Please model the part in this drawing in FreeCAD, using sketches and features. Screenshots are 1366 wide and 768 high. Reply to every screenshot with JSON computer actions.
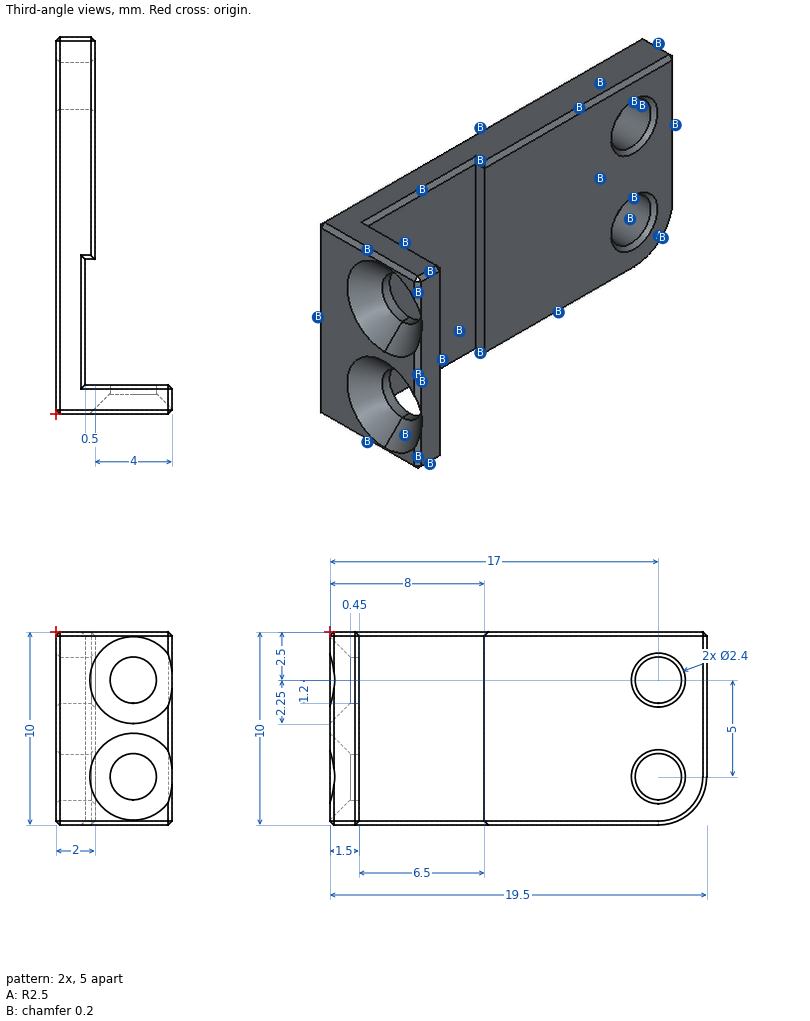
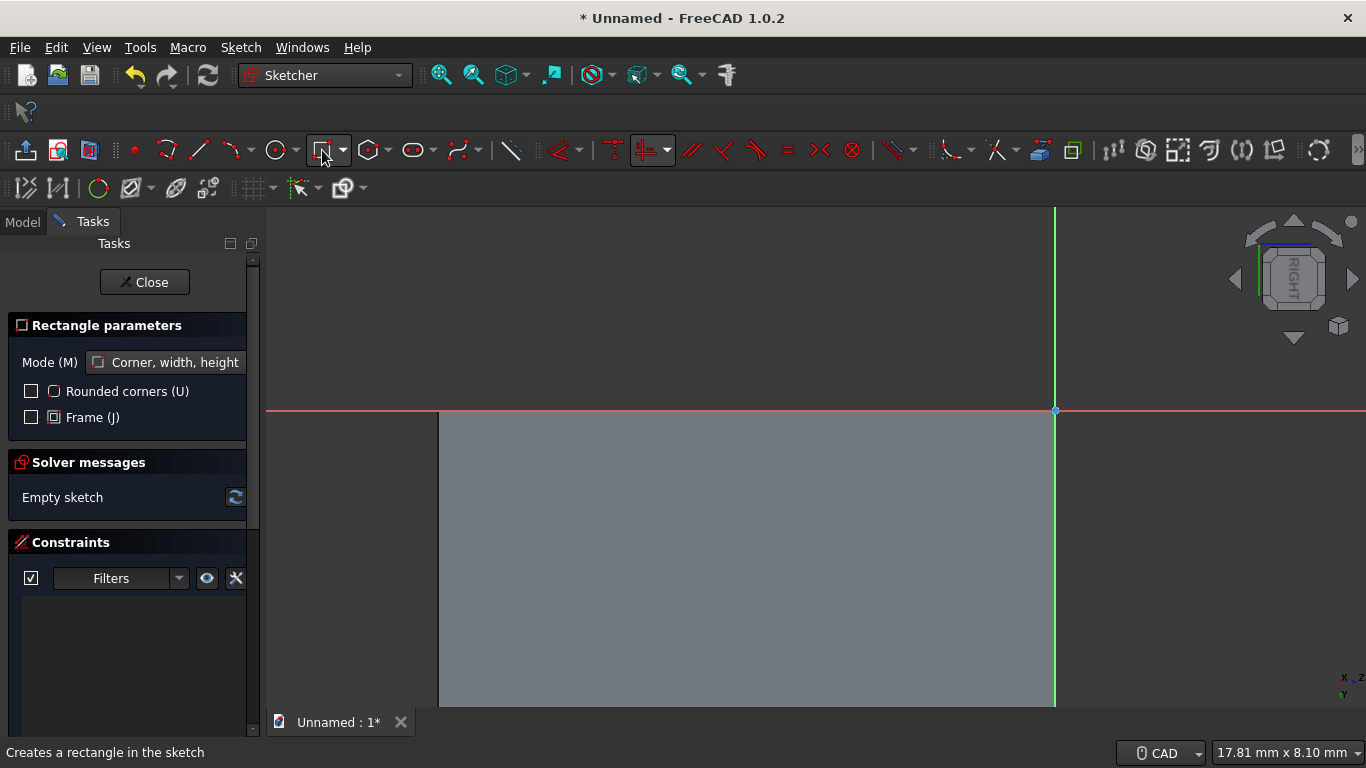
{"action": "left_click", "coordinate": [1055, 411]}
{"action": "left_click", "coordinate": [438, 504]}
{"action": "key", "text": "Escape"}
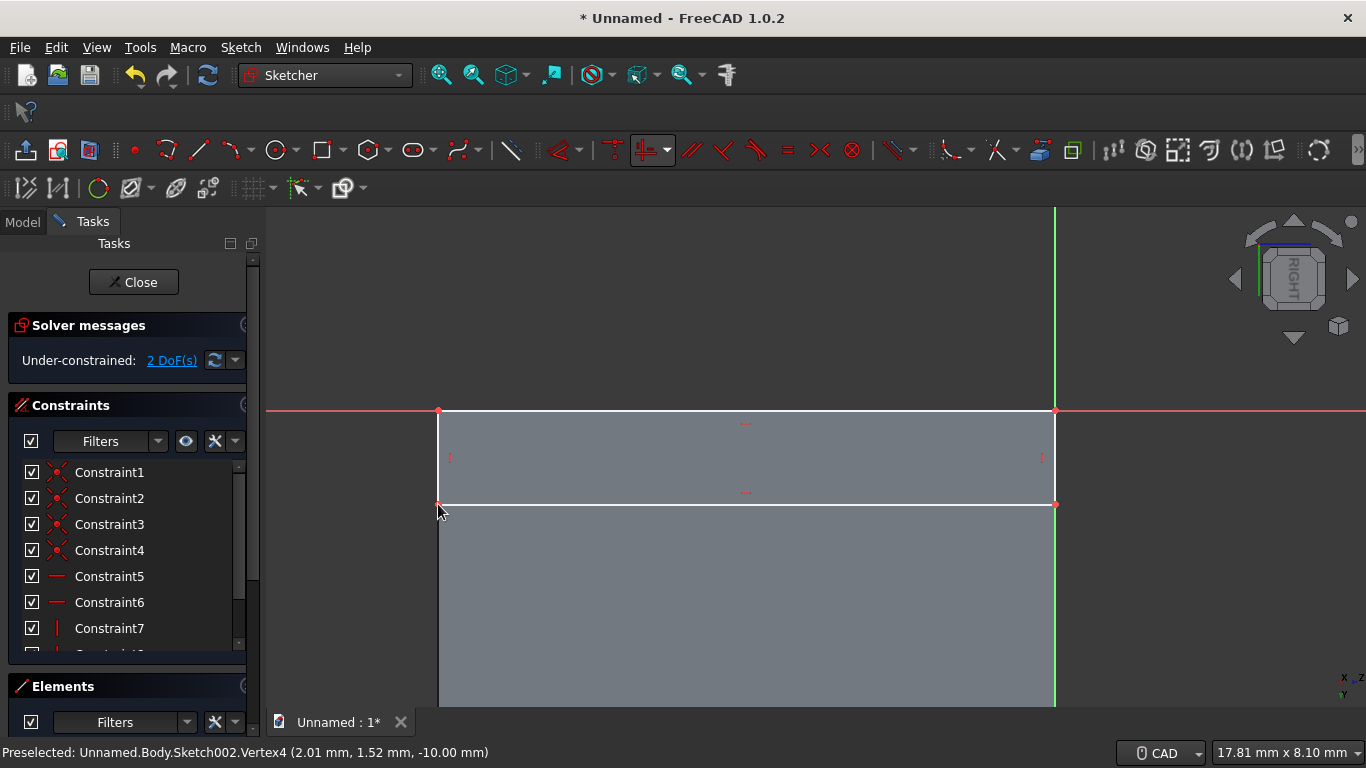
{"action": "left_click", "coordinate": [558, 150]}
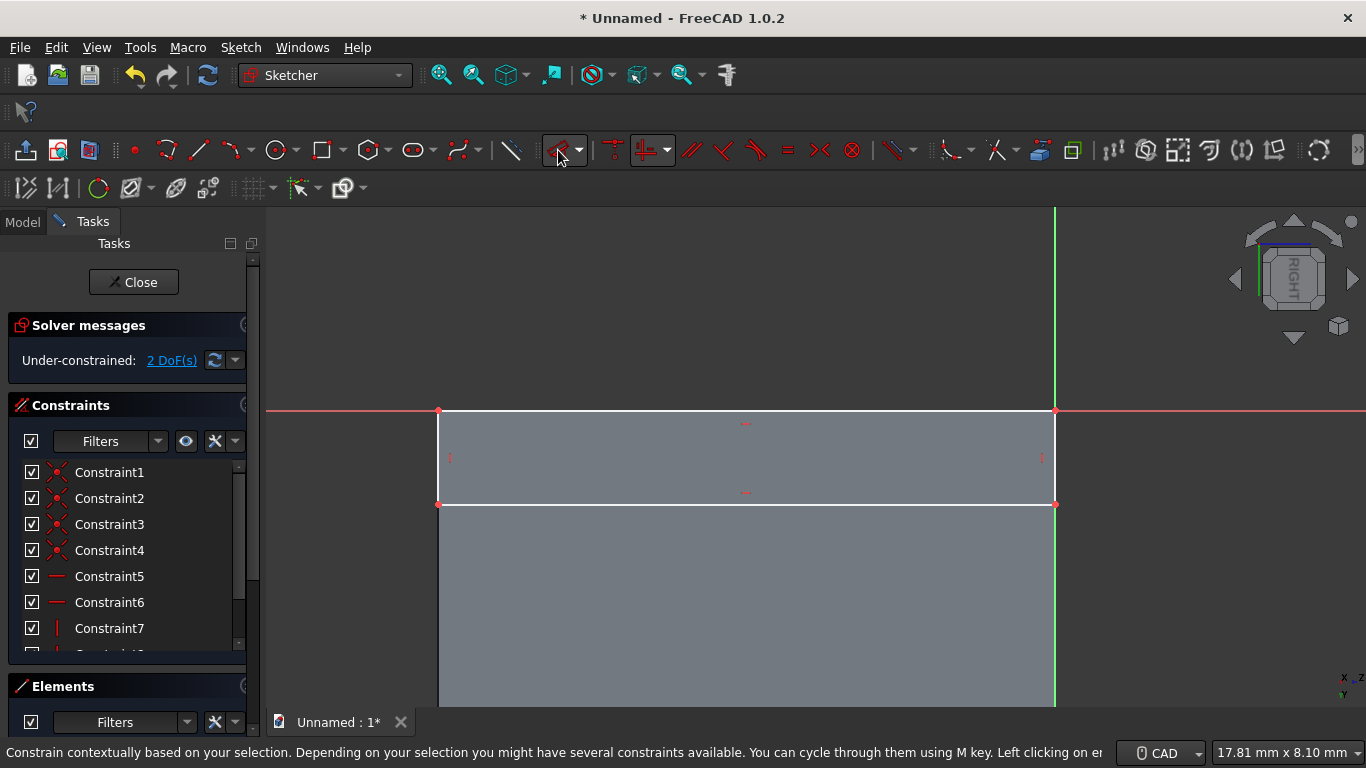
{"action": "left_click", "coordinate": [870, 411]}
{"action": "left_click", "coordinate": [747, 377]}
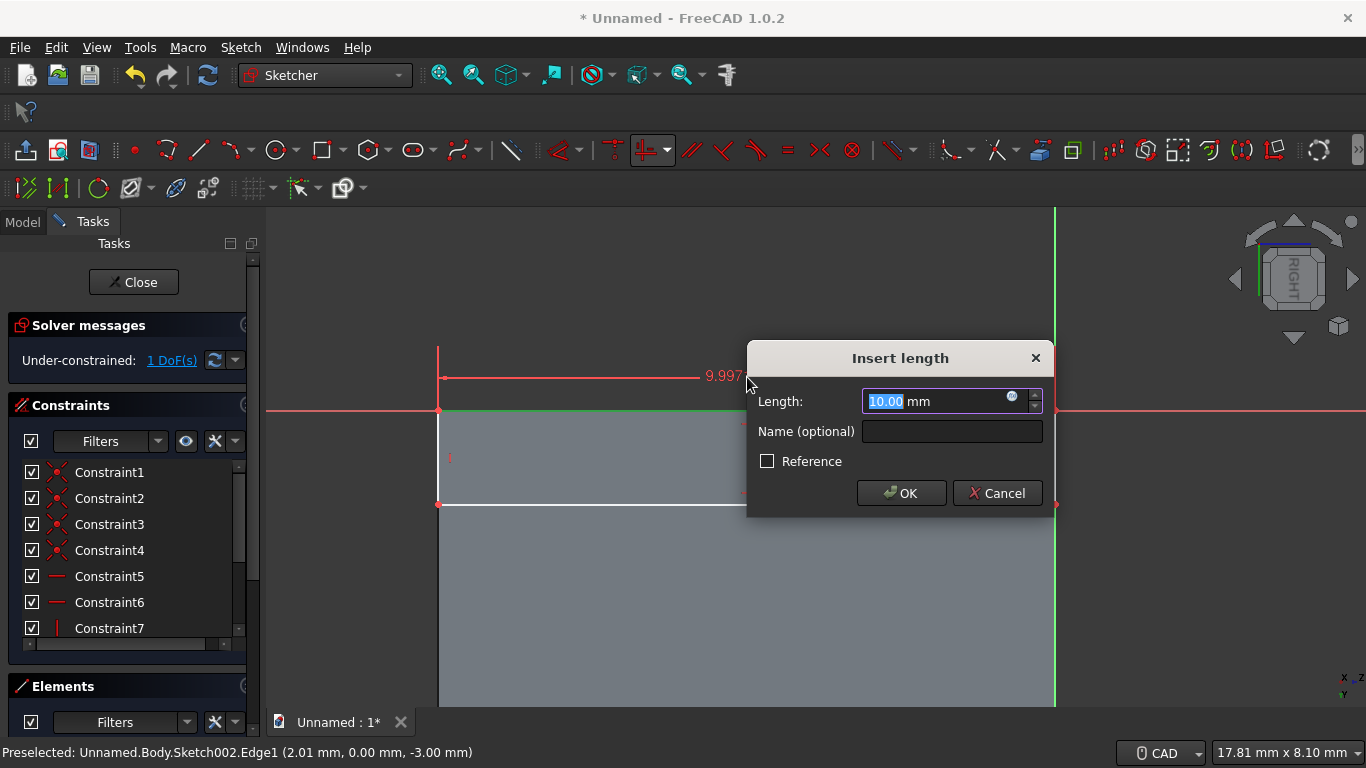
{"action": "type", "text": "10"}
{"action": "key", "text": "Return"}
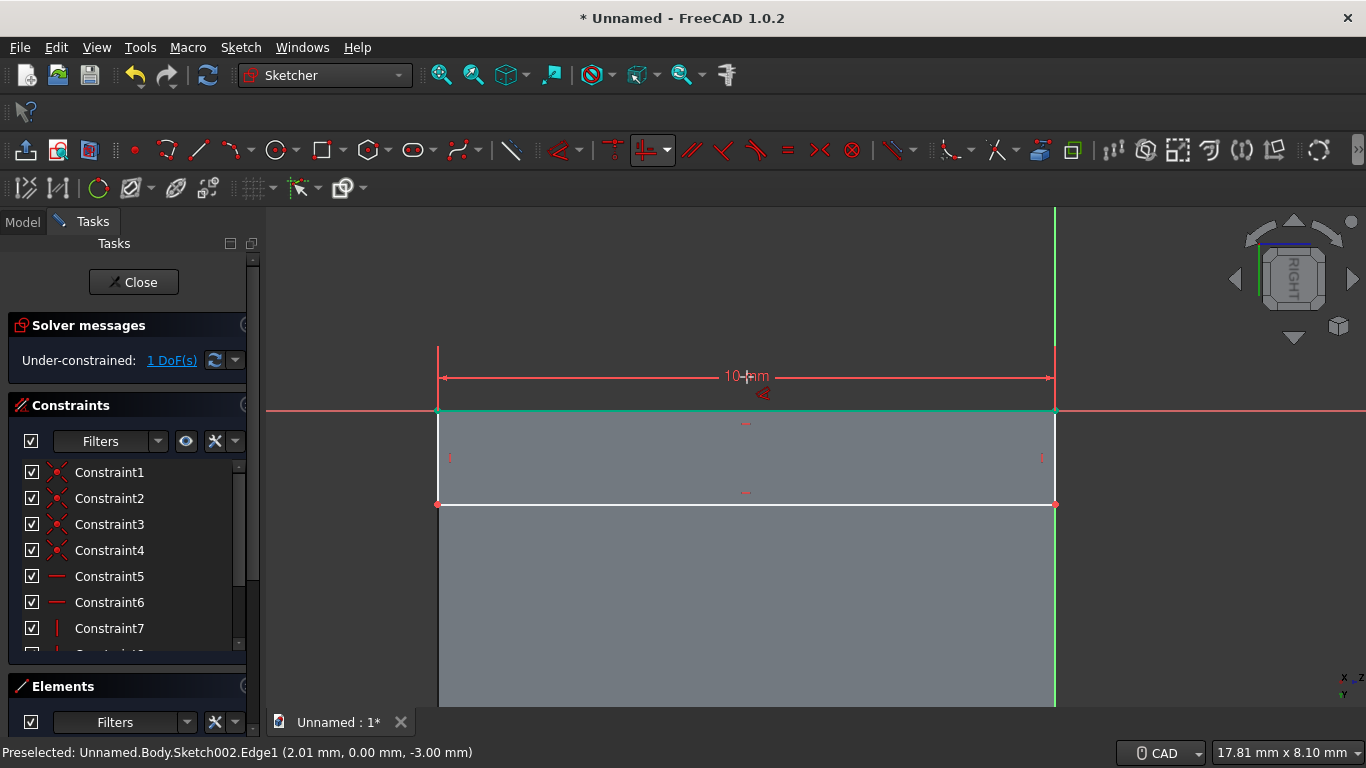
{"action": "left_click", "coordinate": [438, 439]}
{"action": "left_click", "coordinate": [404, 458]}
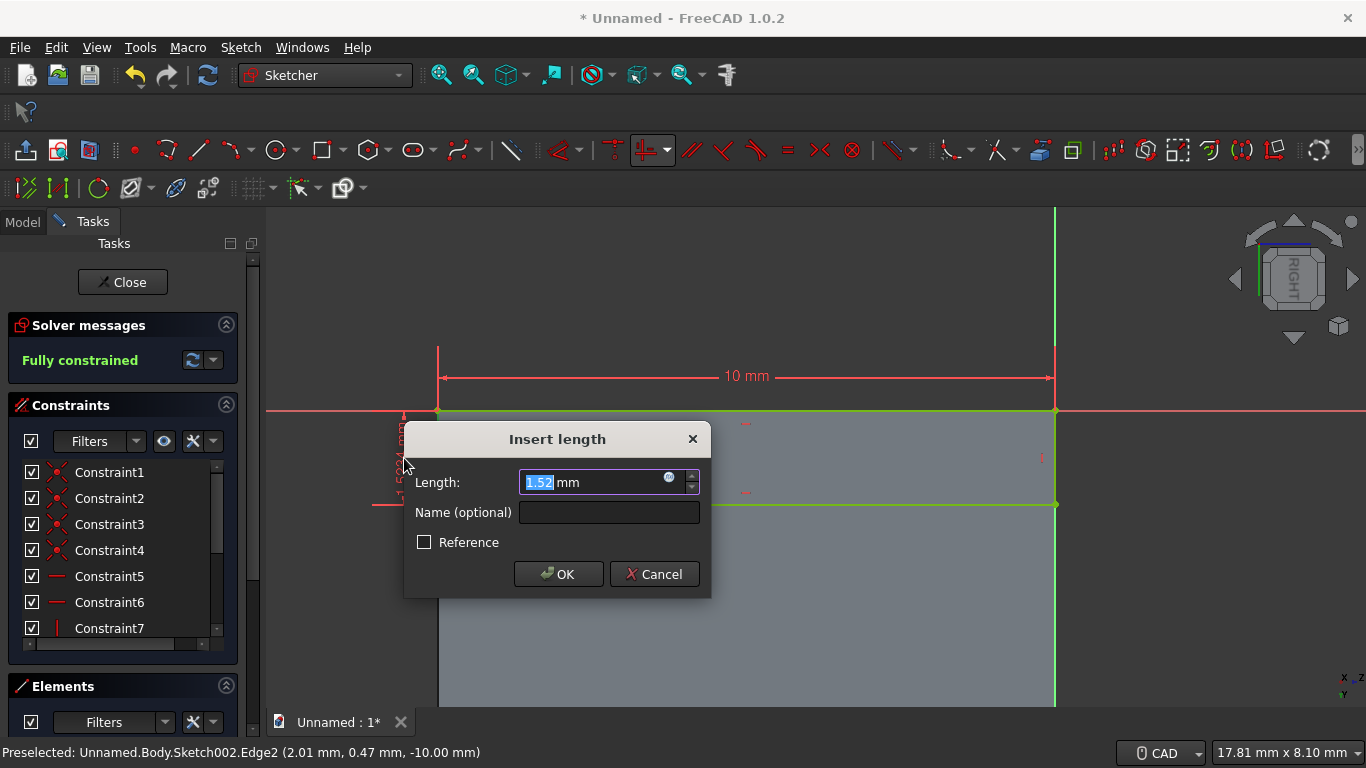
{"action": "type", "text": "1.5"}
{"action": "key", "text": "Return"}
{"action": "key", "text": "Escape"}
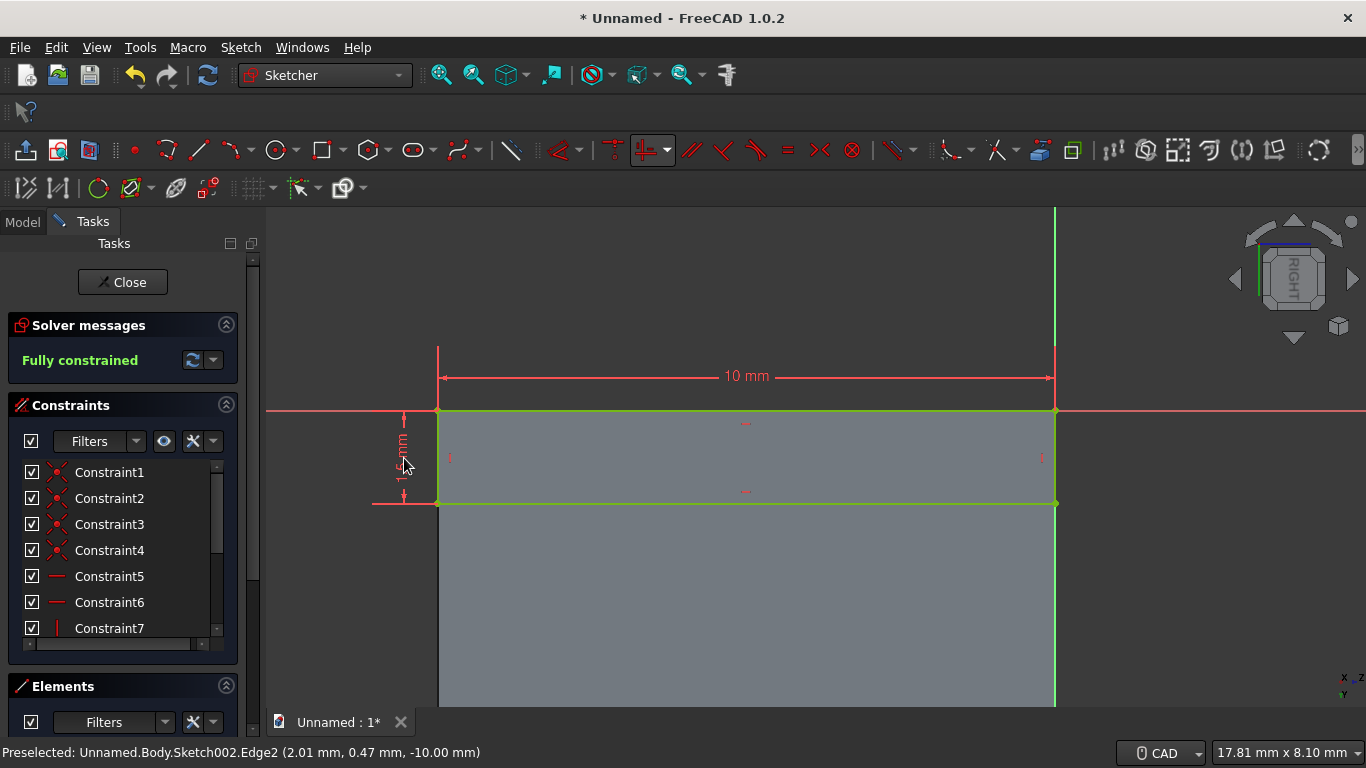
{"action": "left_click", "coordinate": [123, 282]}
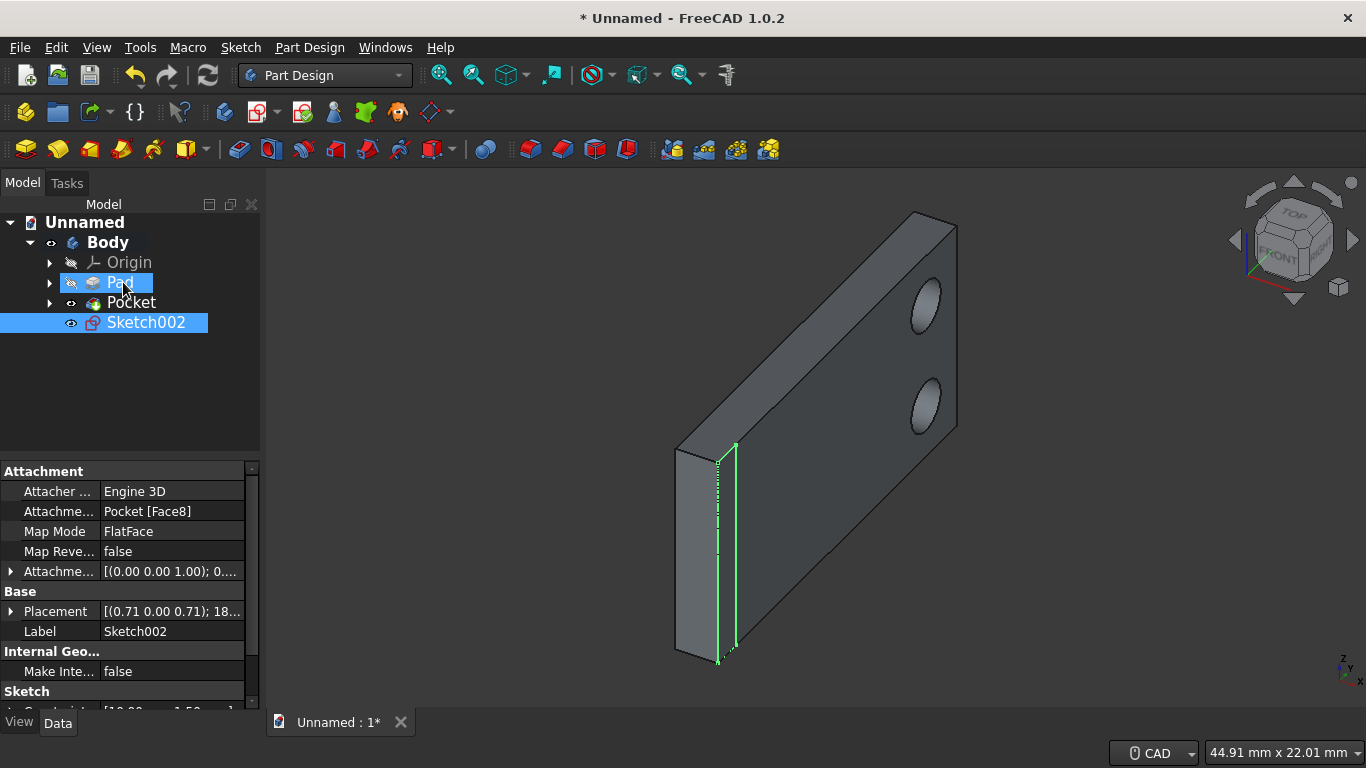
{"action": "left_click", "coordinate": [26, 150]}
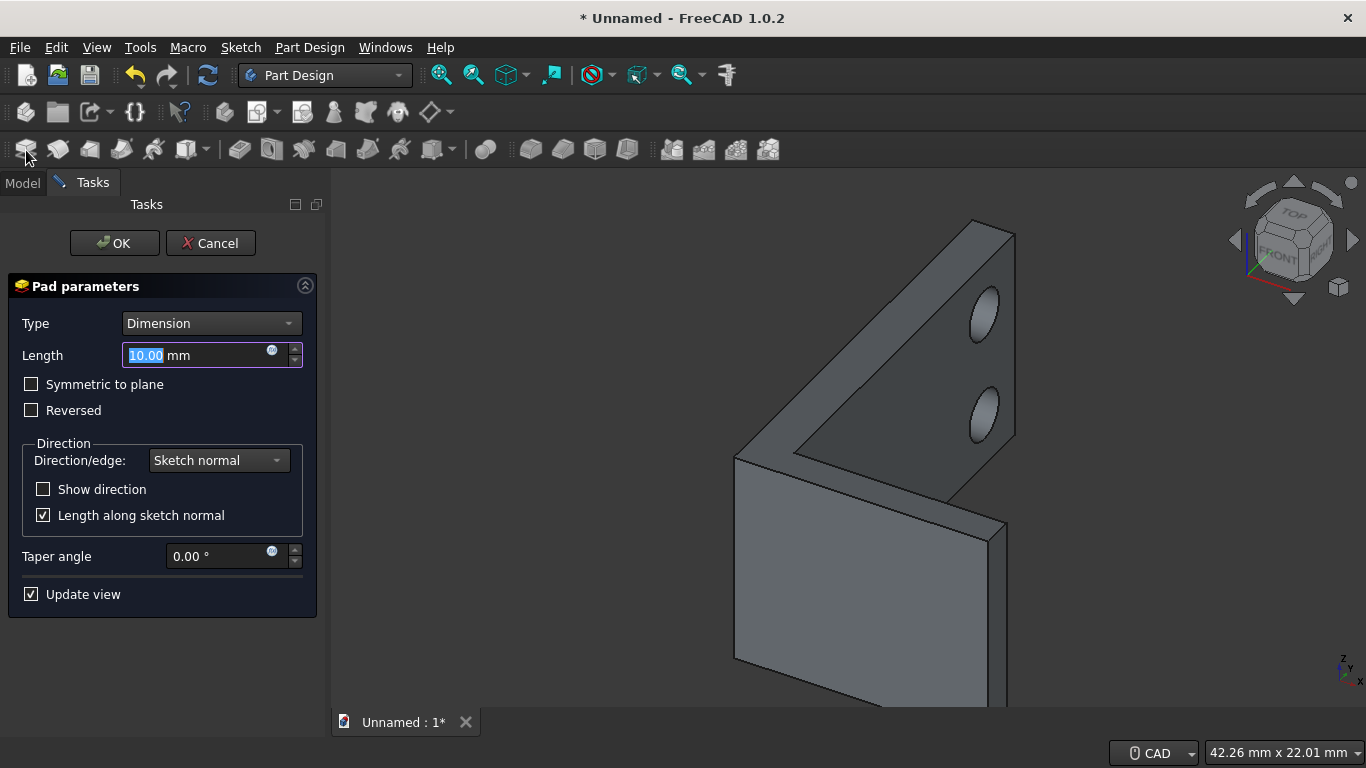
{"action": "type", "text": "4"}
{"action": "key", "text": "Tab"}